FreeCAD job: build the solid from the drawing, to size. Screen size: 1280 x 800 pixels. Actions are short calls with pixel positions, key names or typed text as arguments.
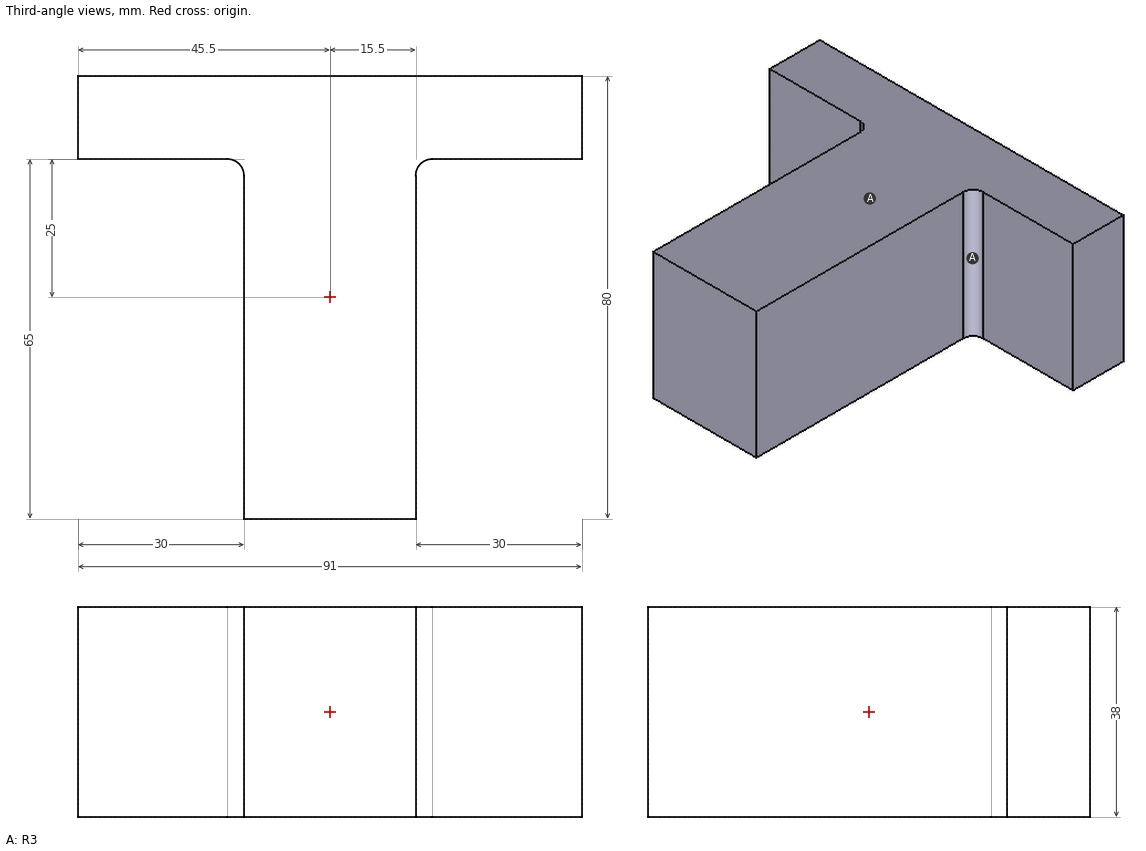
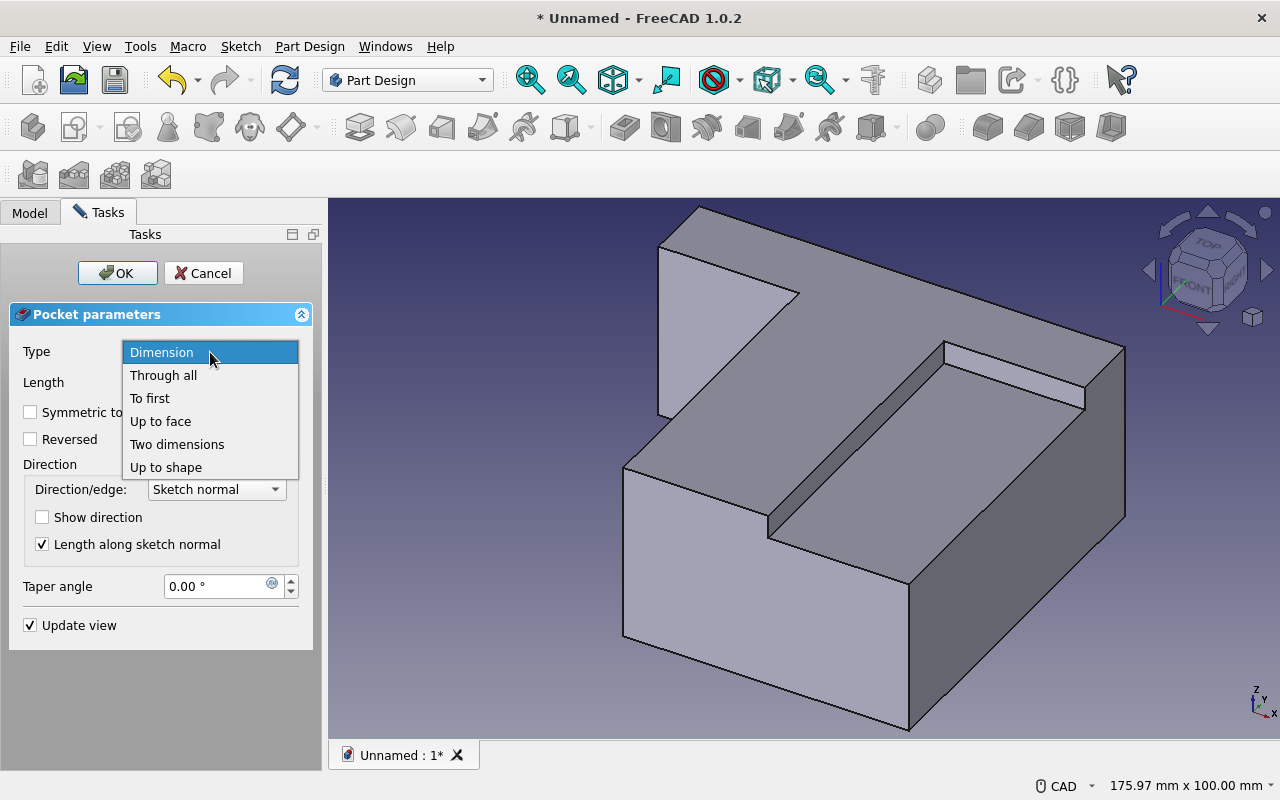
click(208, 398)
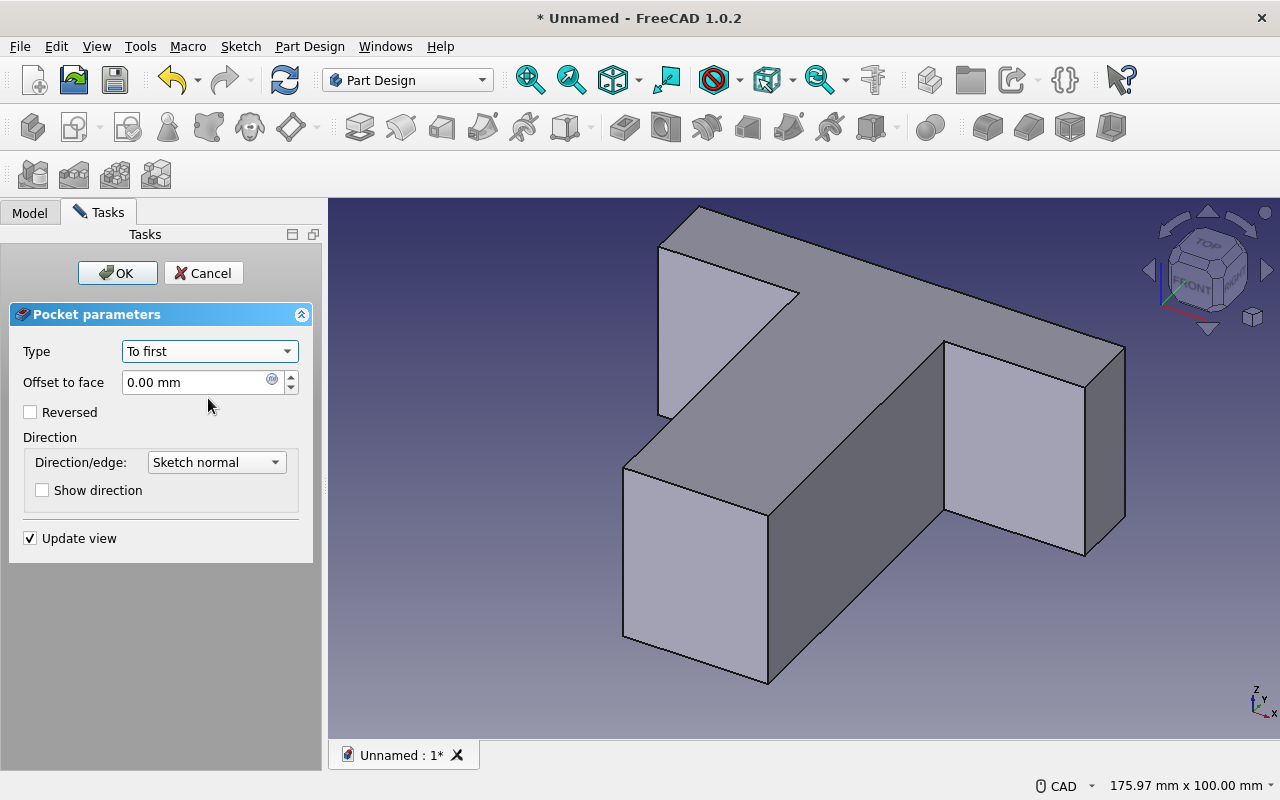
click(118, 273)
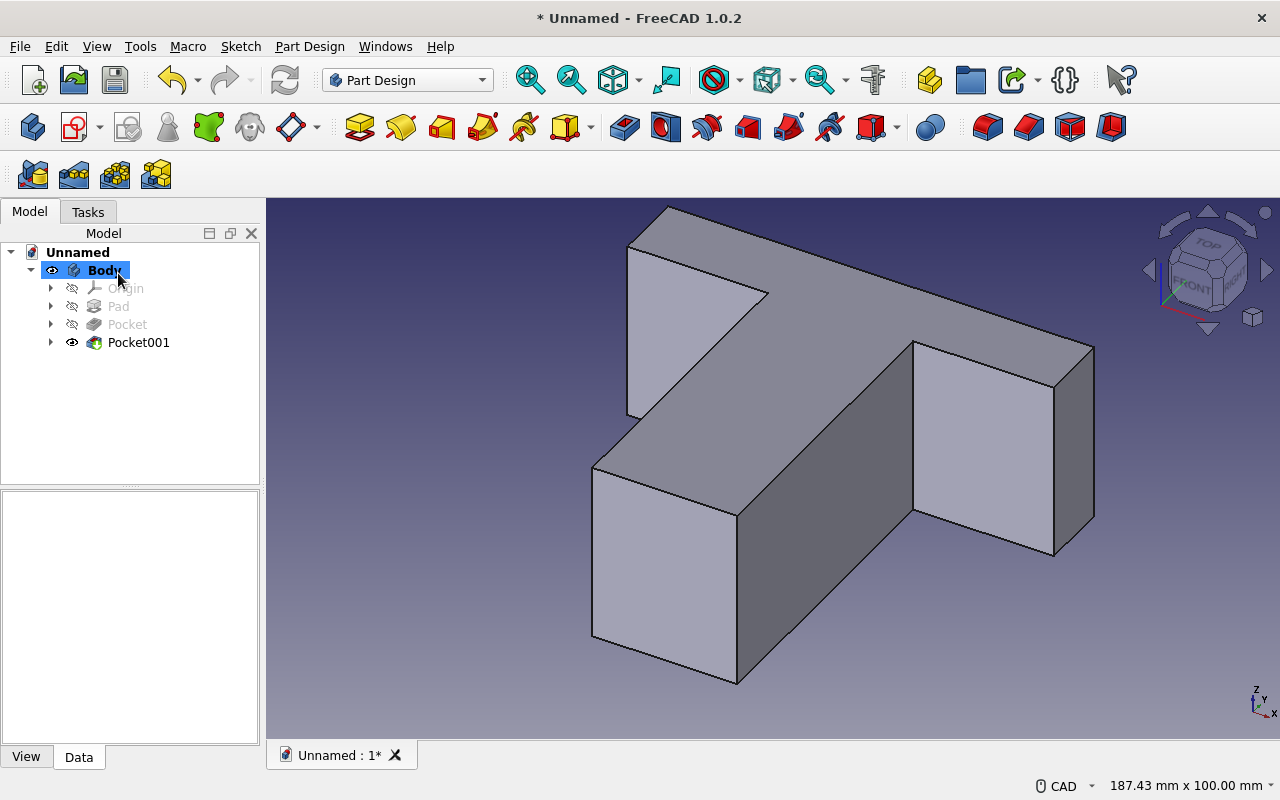
key(0)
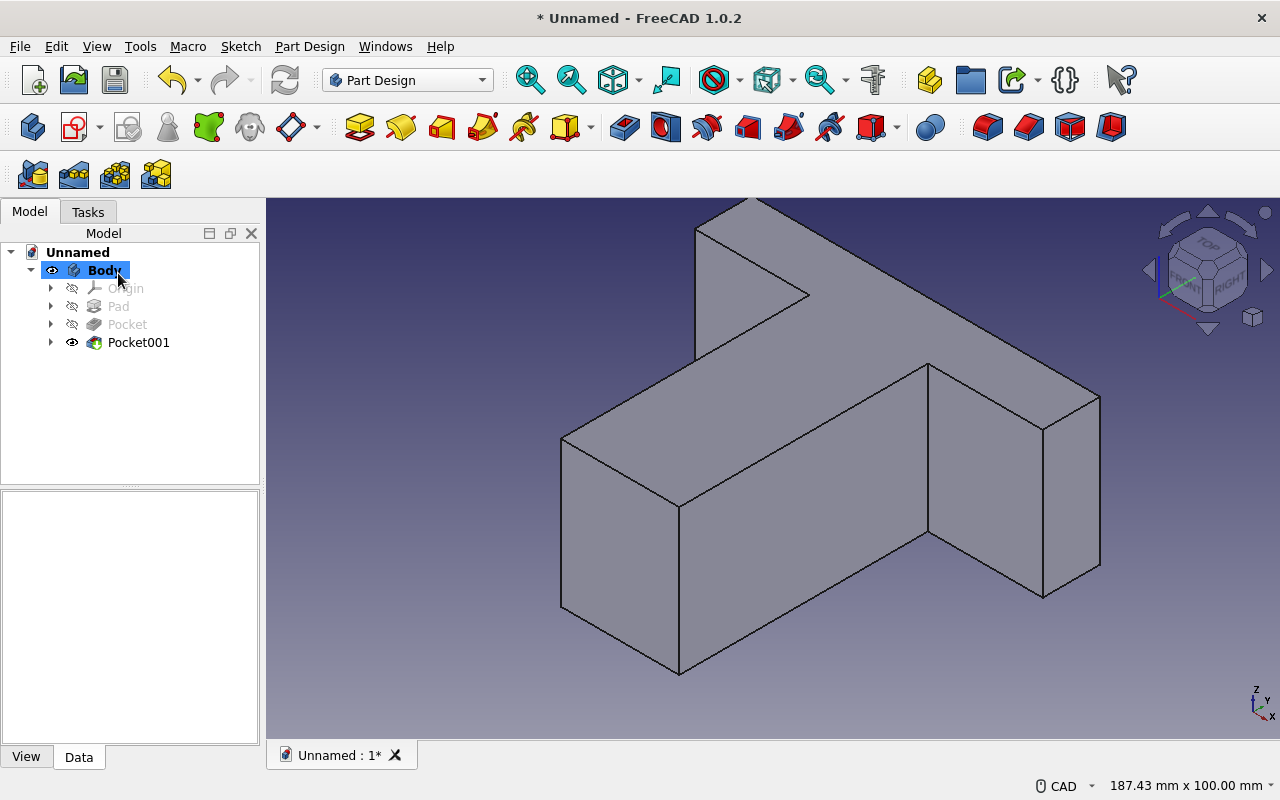
click(531, 80)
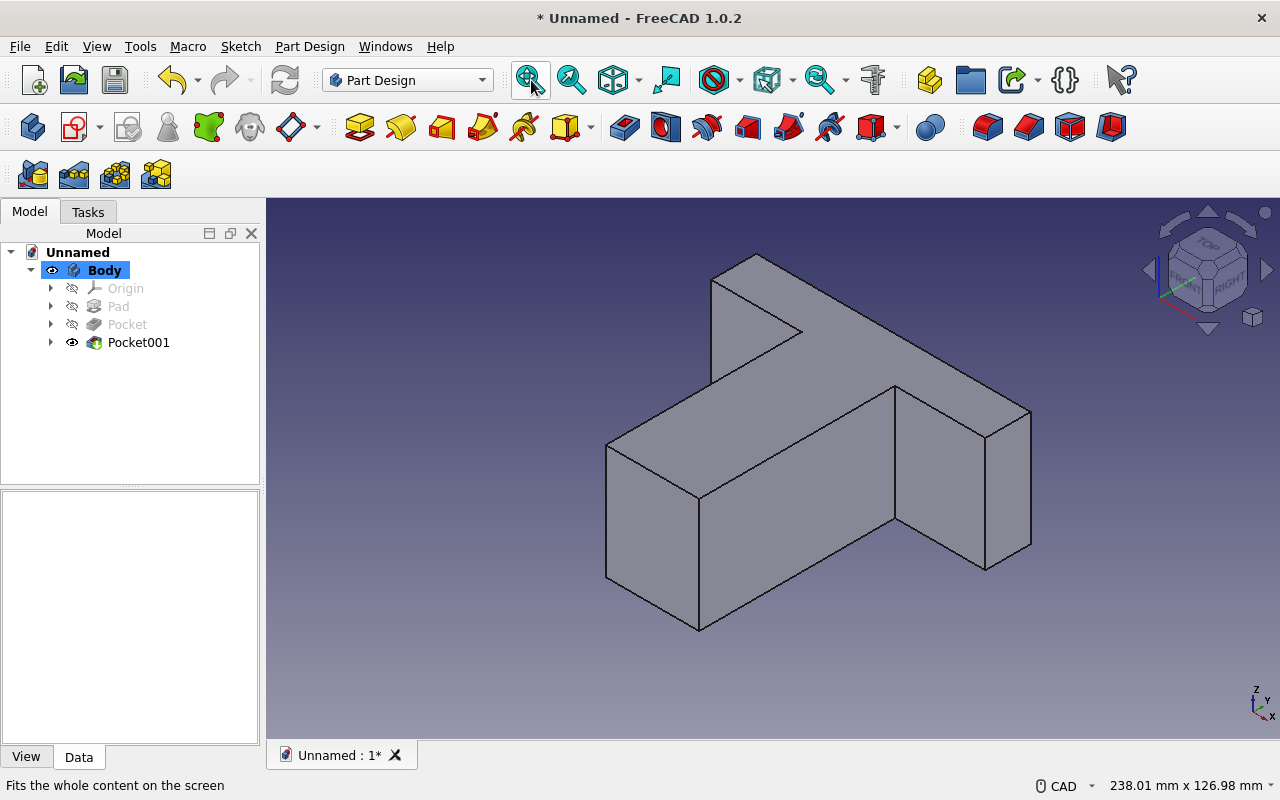
key(2)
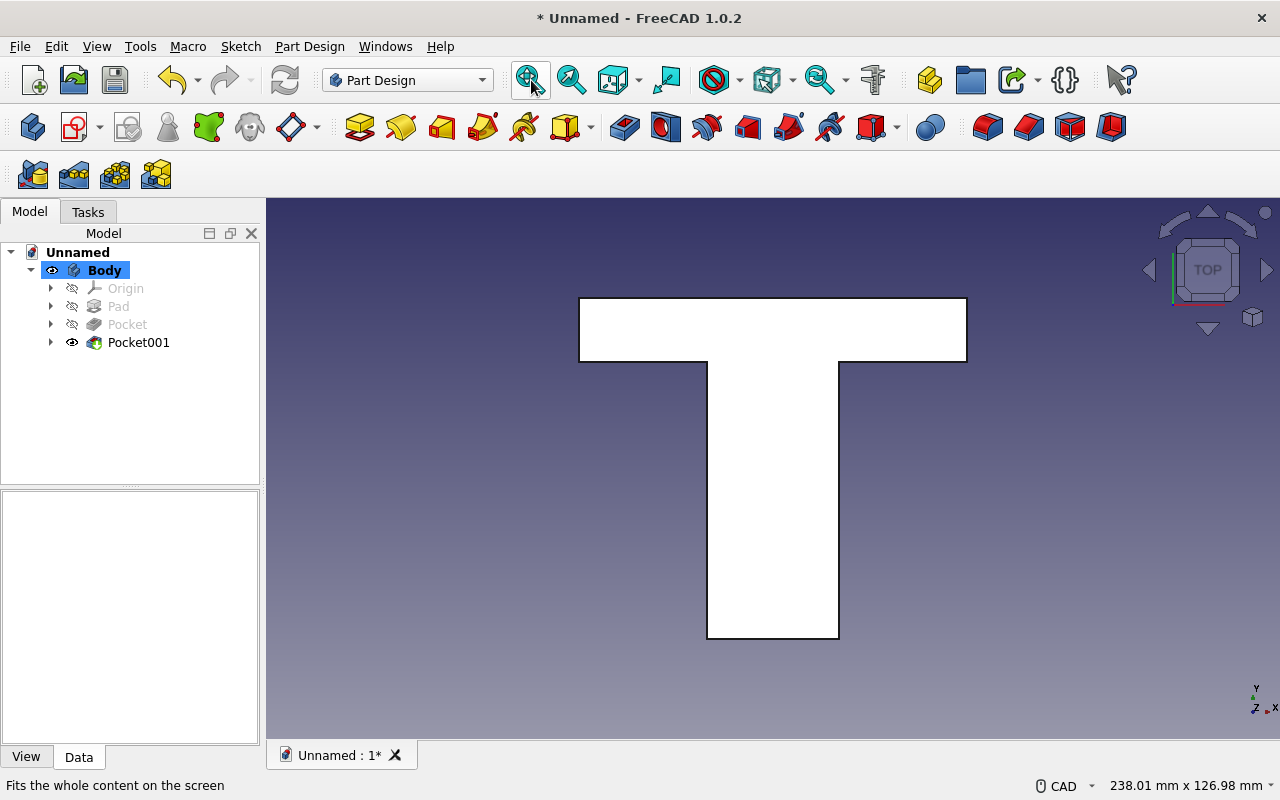
key(1)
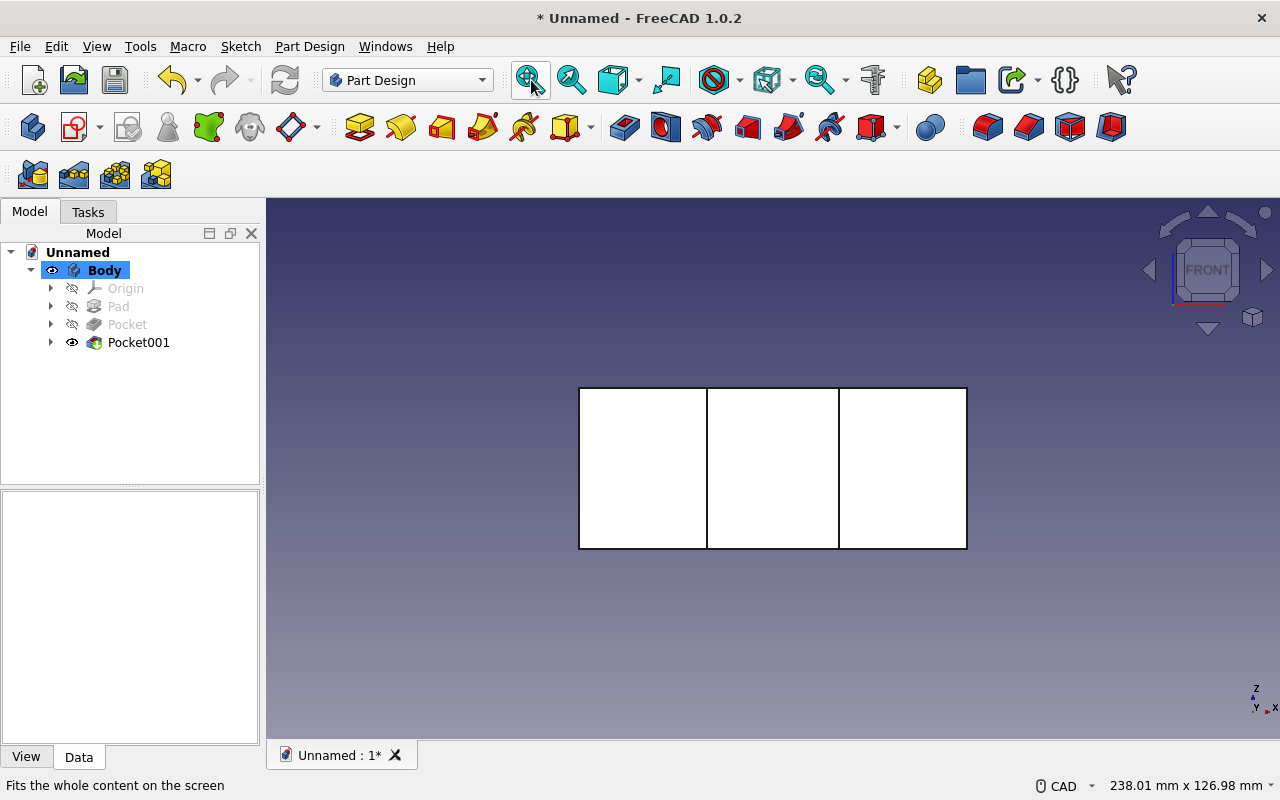
click(531, 80)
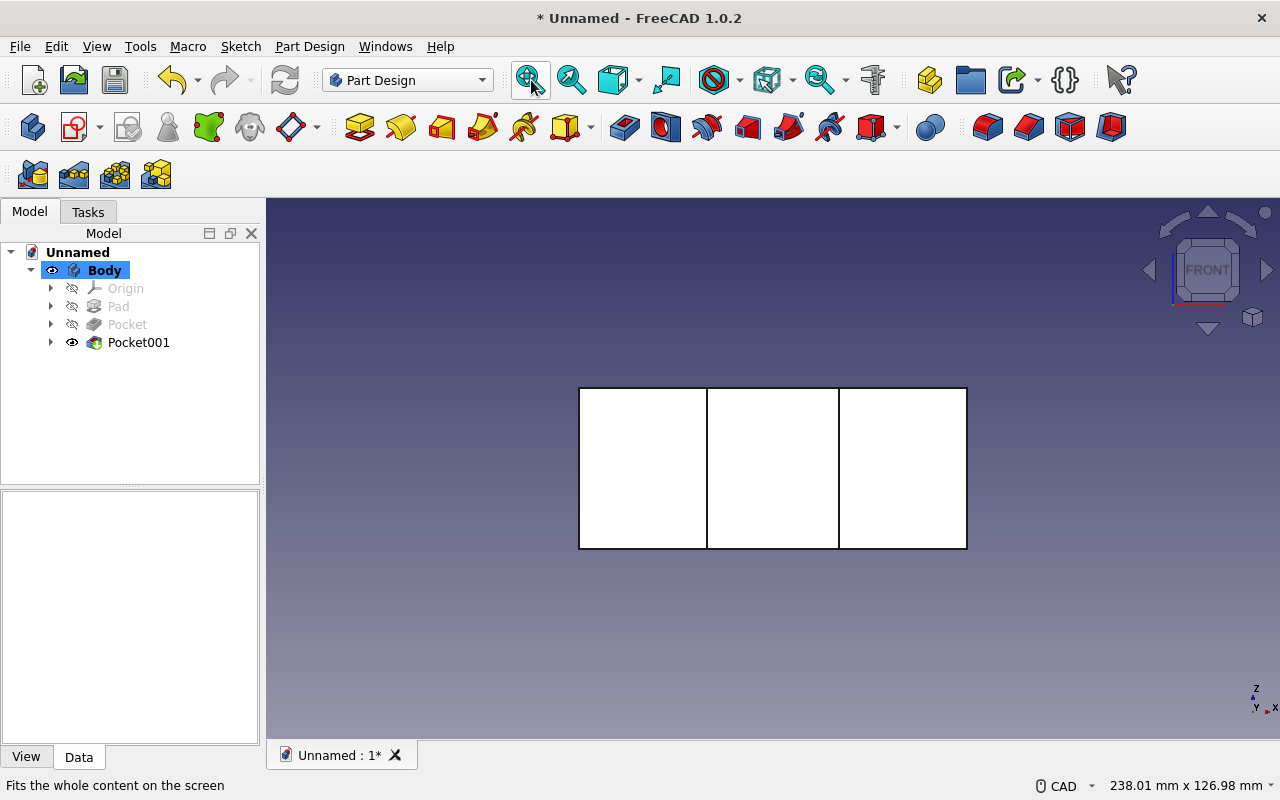
key(3)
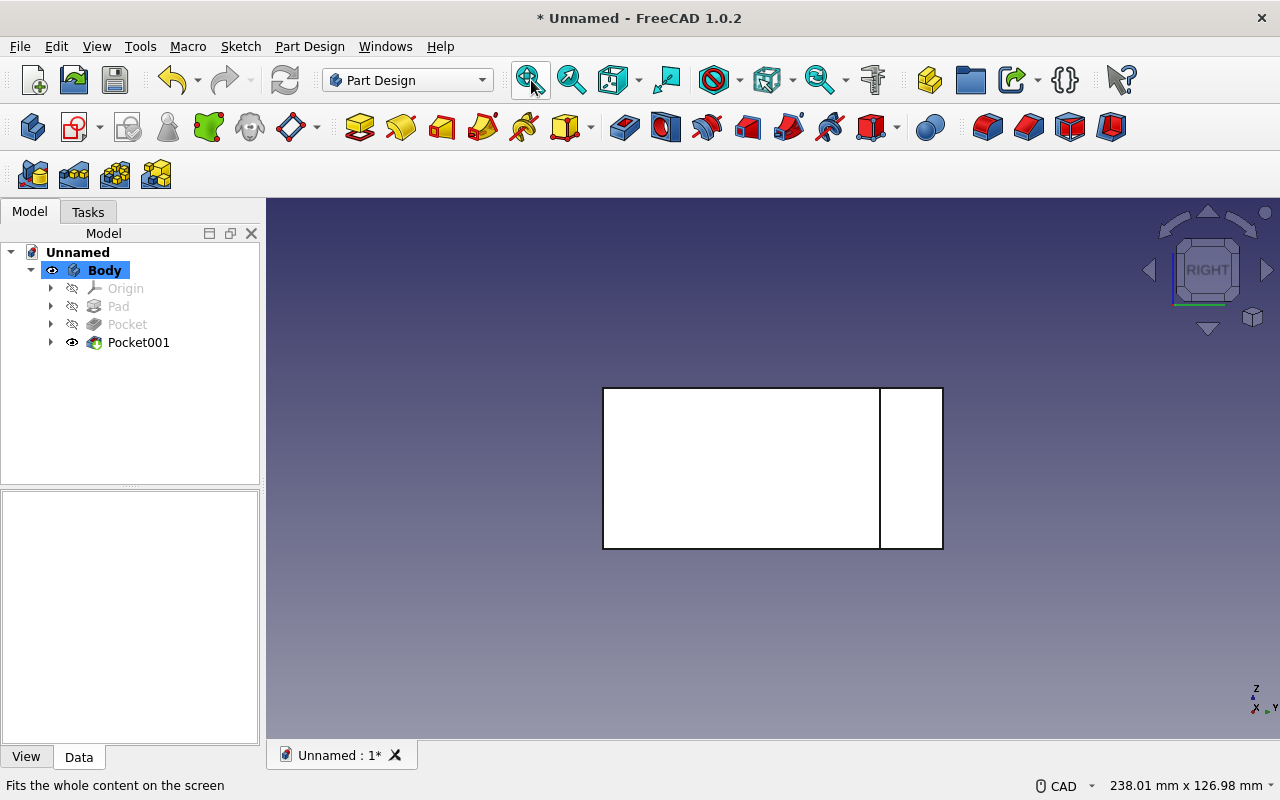
click(531, 80)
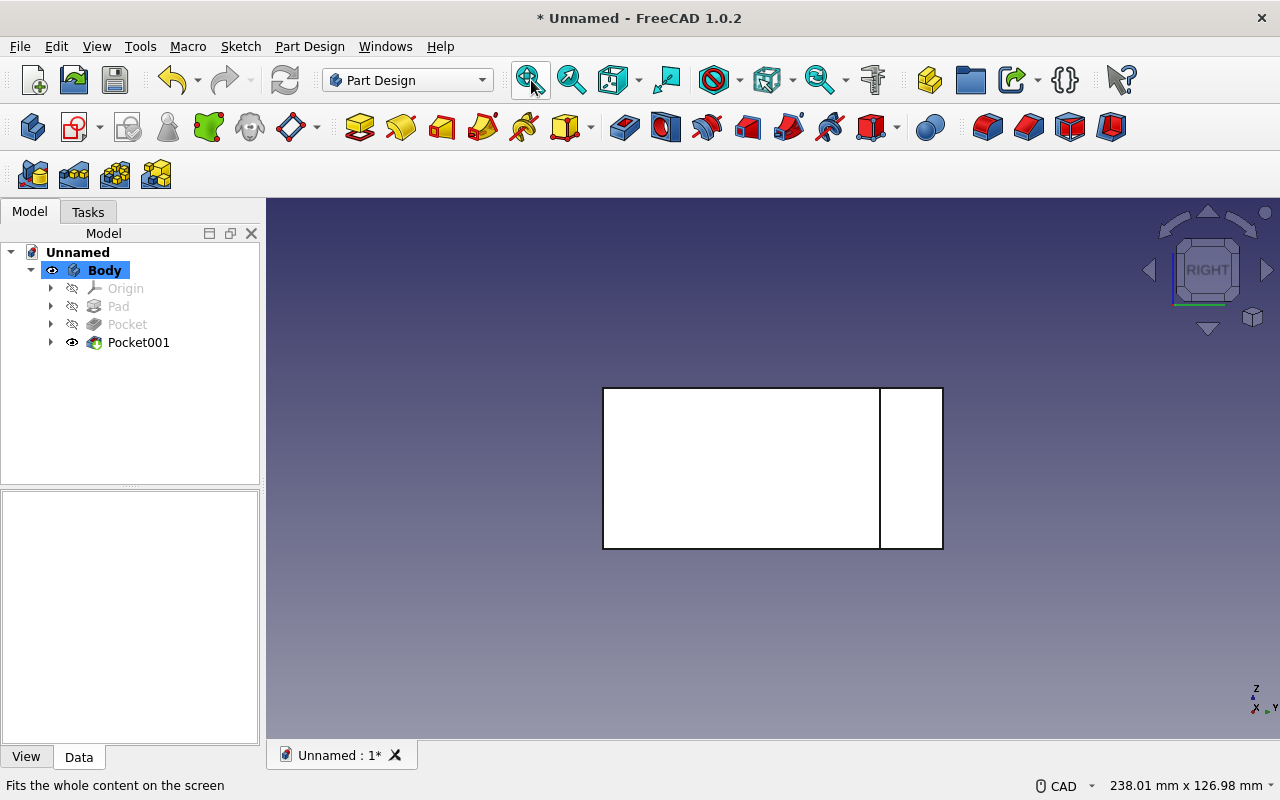
key(5)